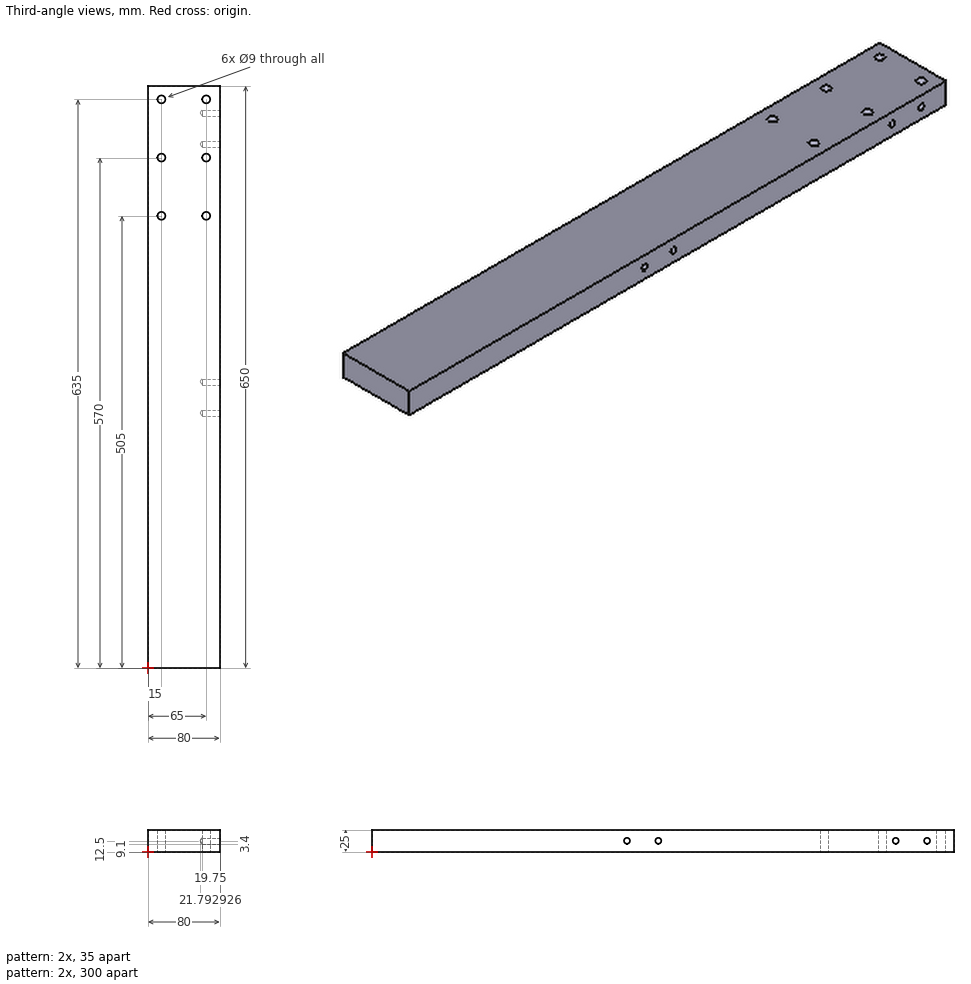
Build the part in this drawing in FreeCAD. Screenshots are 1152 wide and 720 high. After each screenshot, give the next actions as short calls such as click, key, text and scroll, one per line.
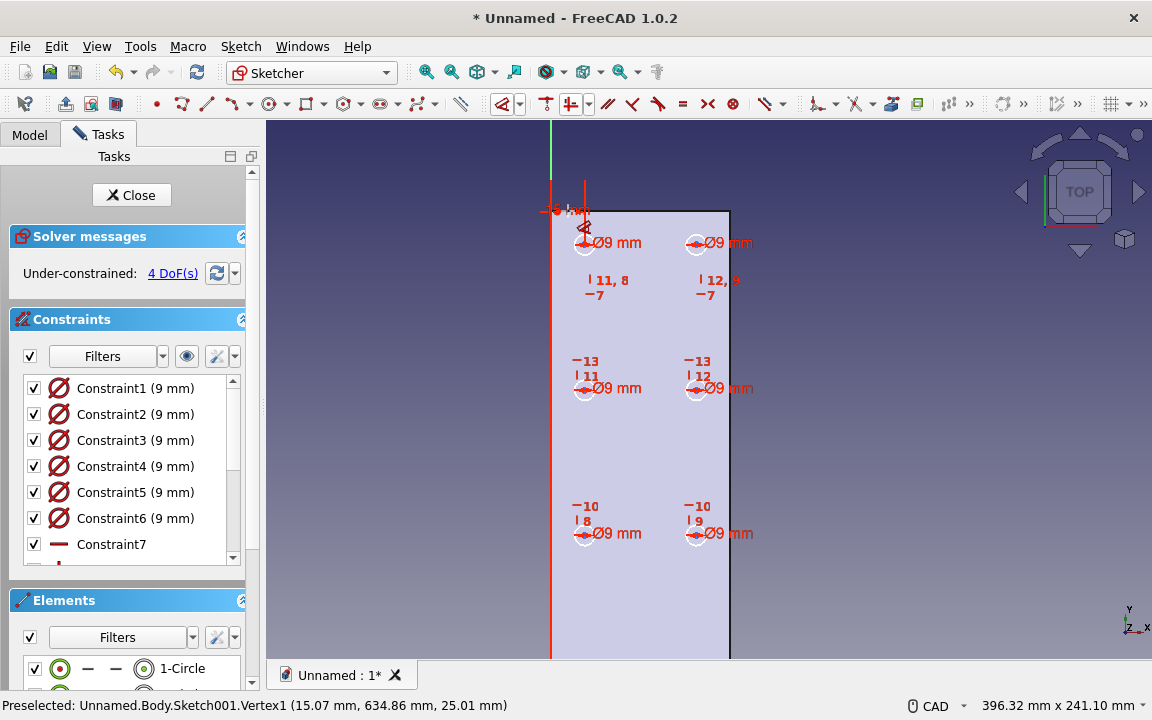
click(696, 245)
click(657, 211)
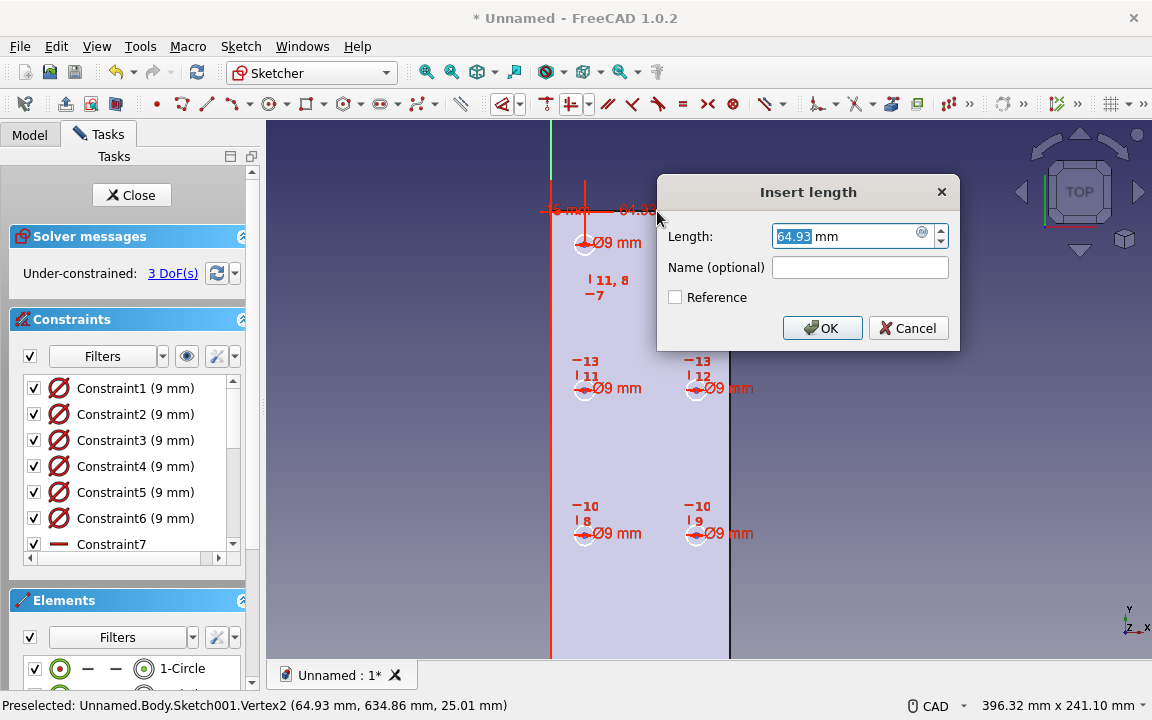
text(65)
key(Return)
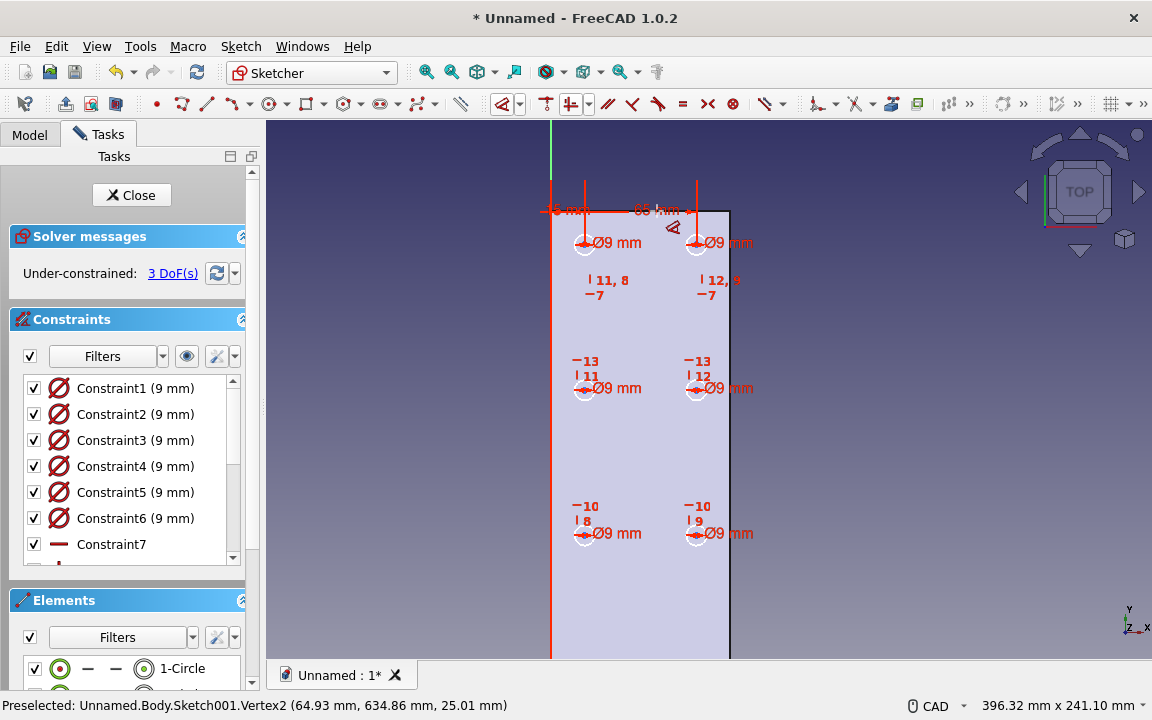
click(585, 245)
click(517, 438)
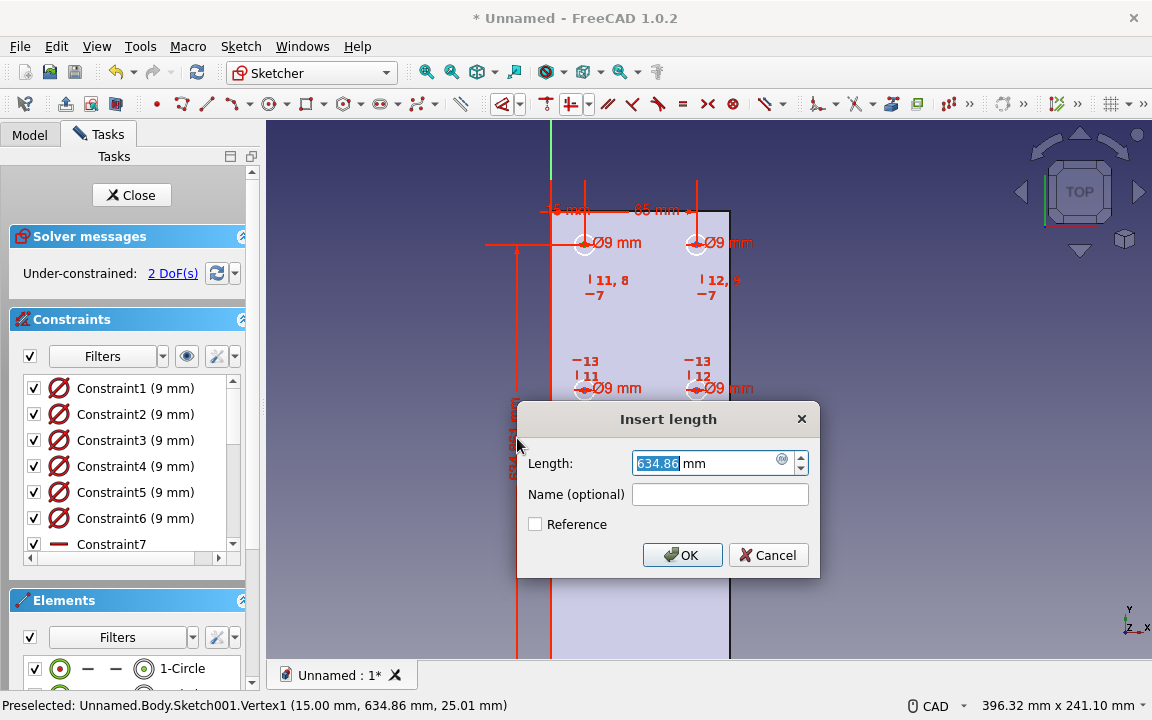
text(635)
key(Return)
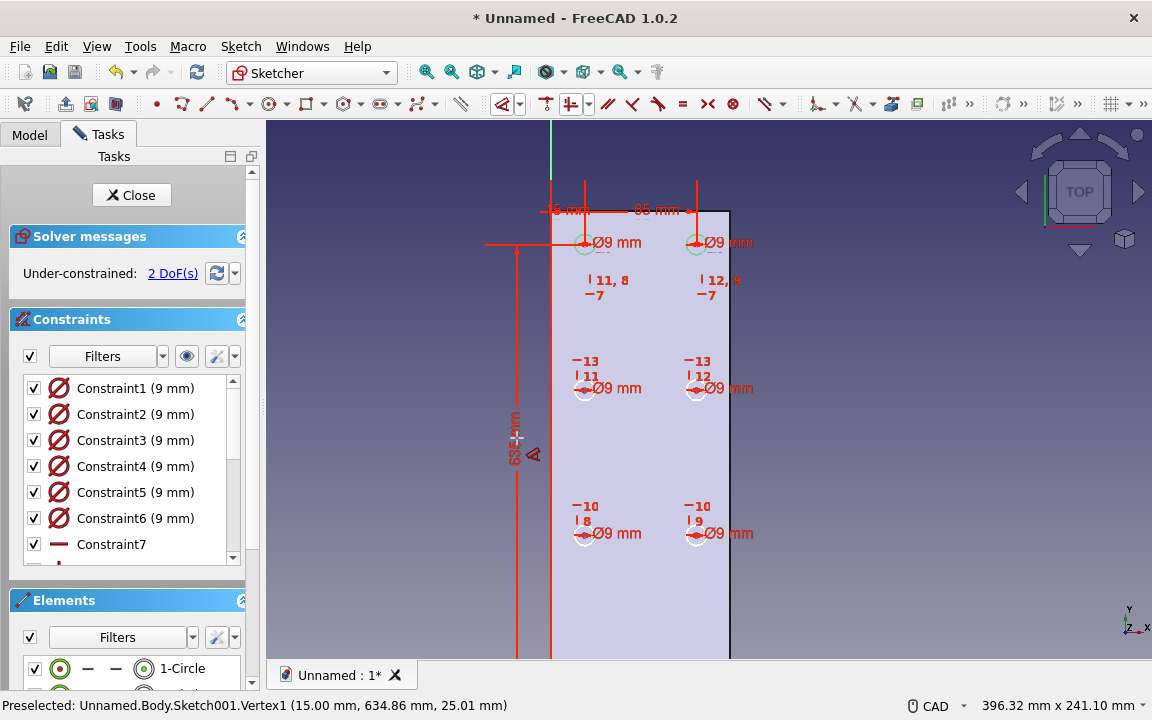
click(585, 535)
click(517, 583)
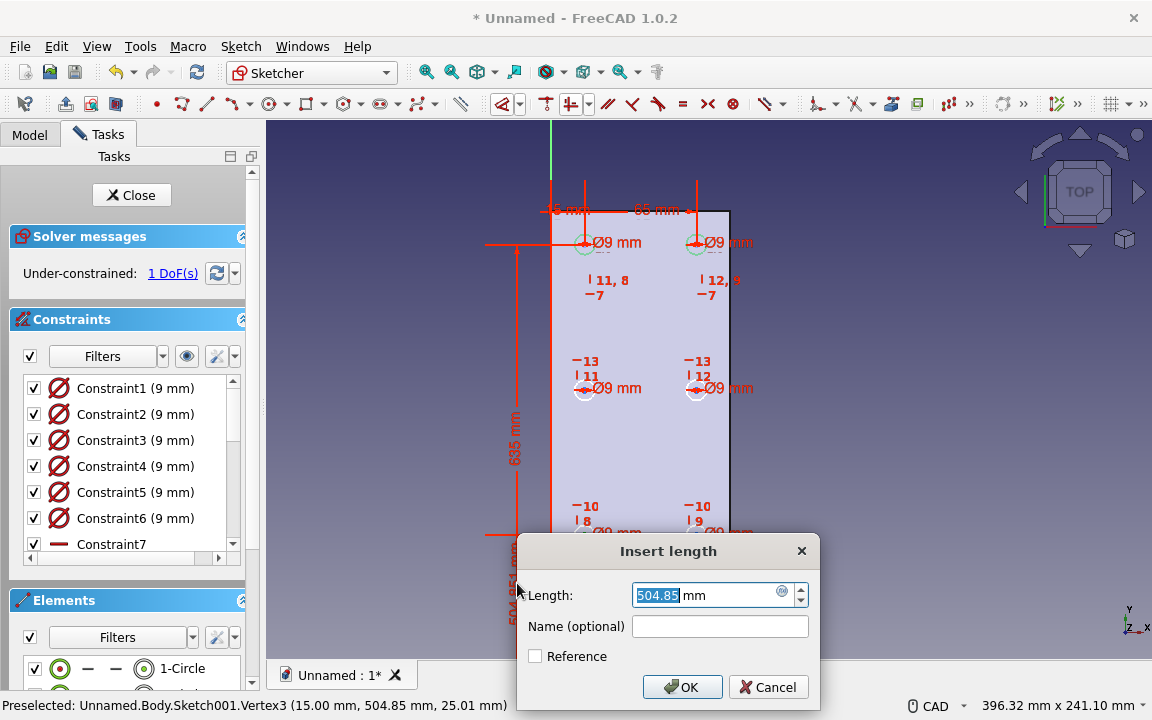
text(505)
key(Return)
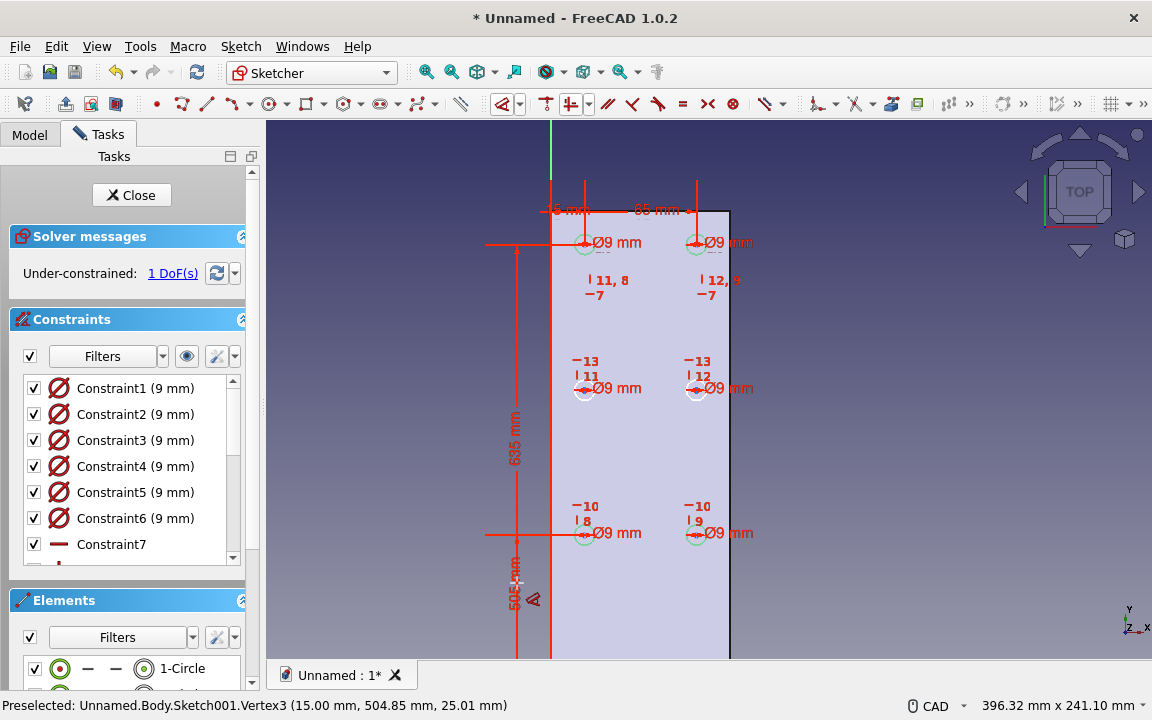
click(585, 390)
click(517, 511)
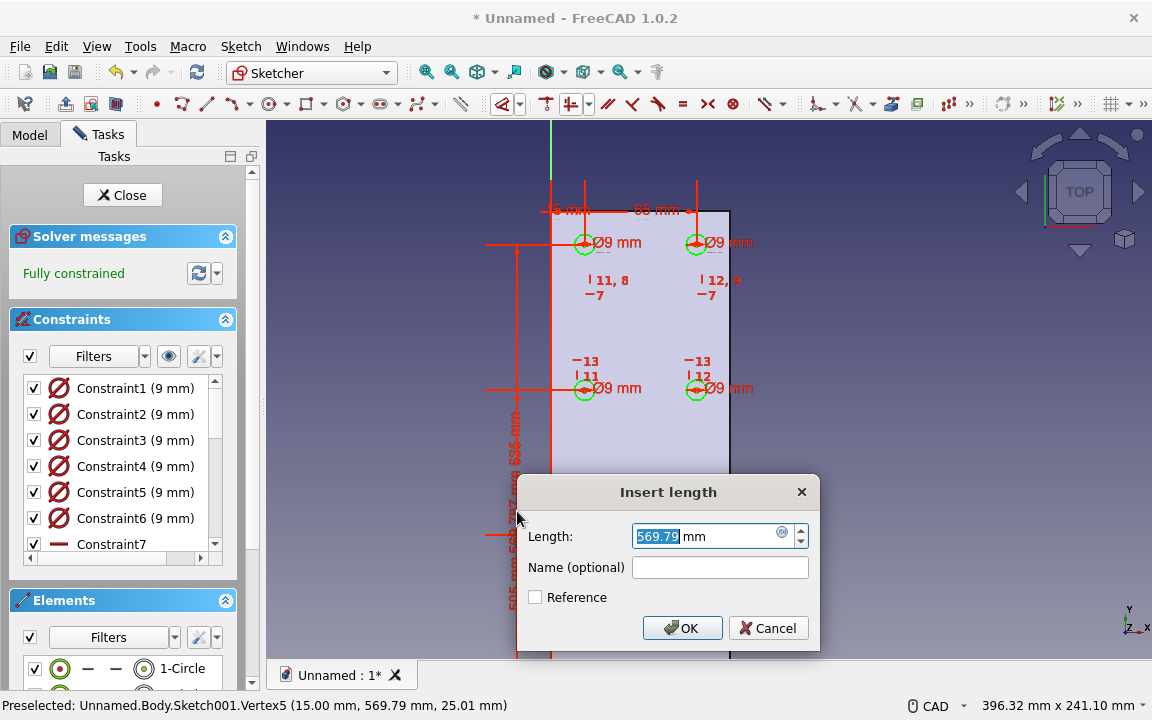
text(570)
key(Return)
key(Escape)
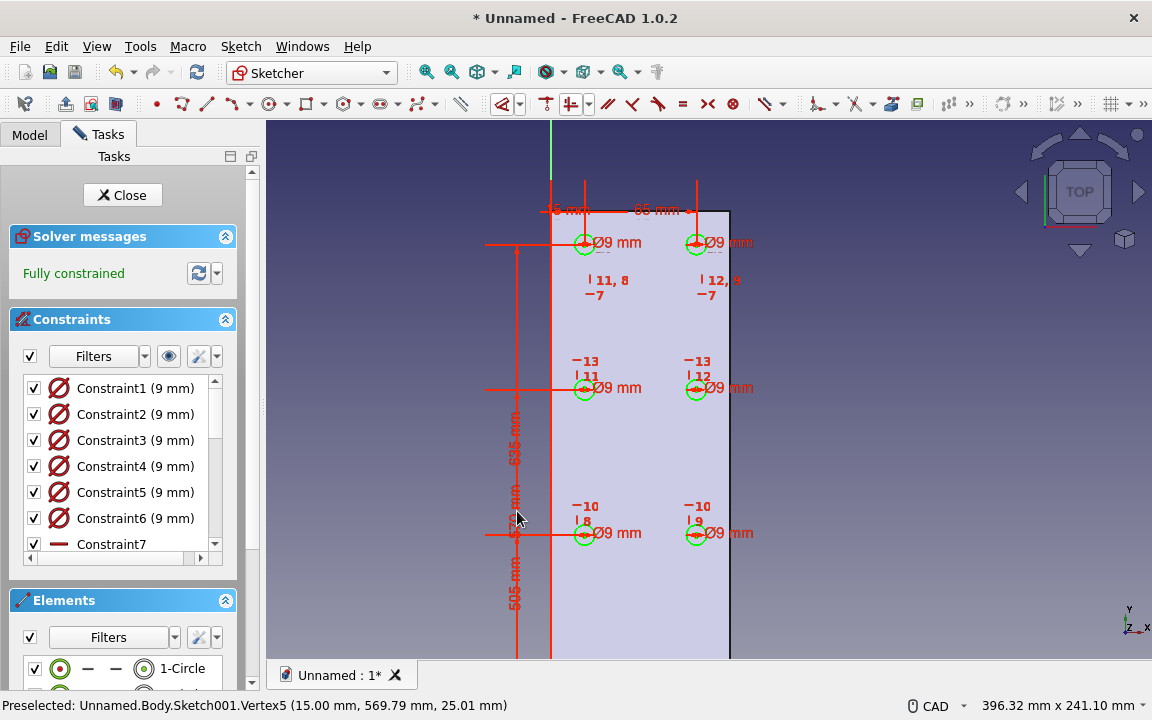
click(123, 195)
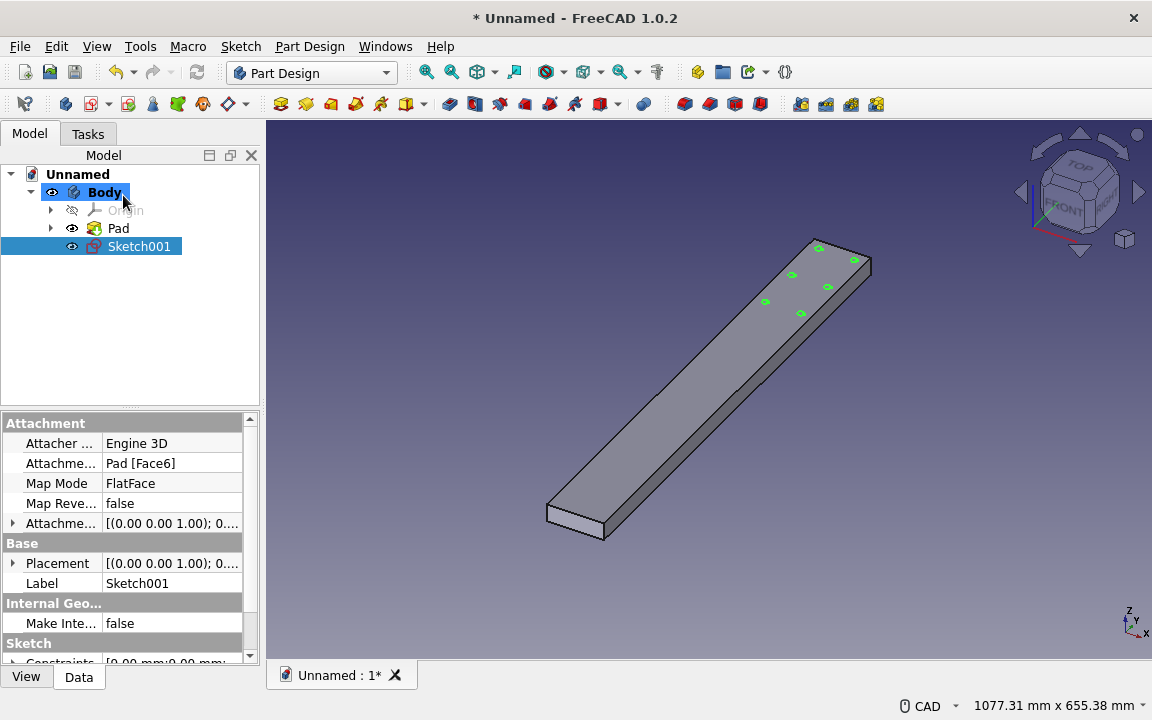
click(475, 104)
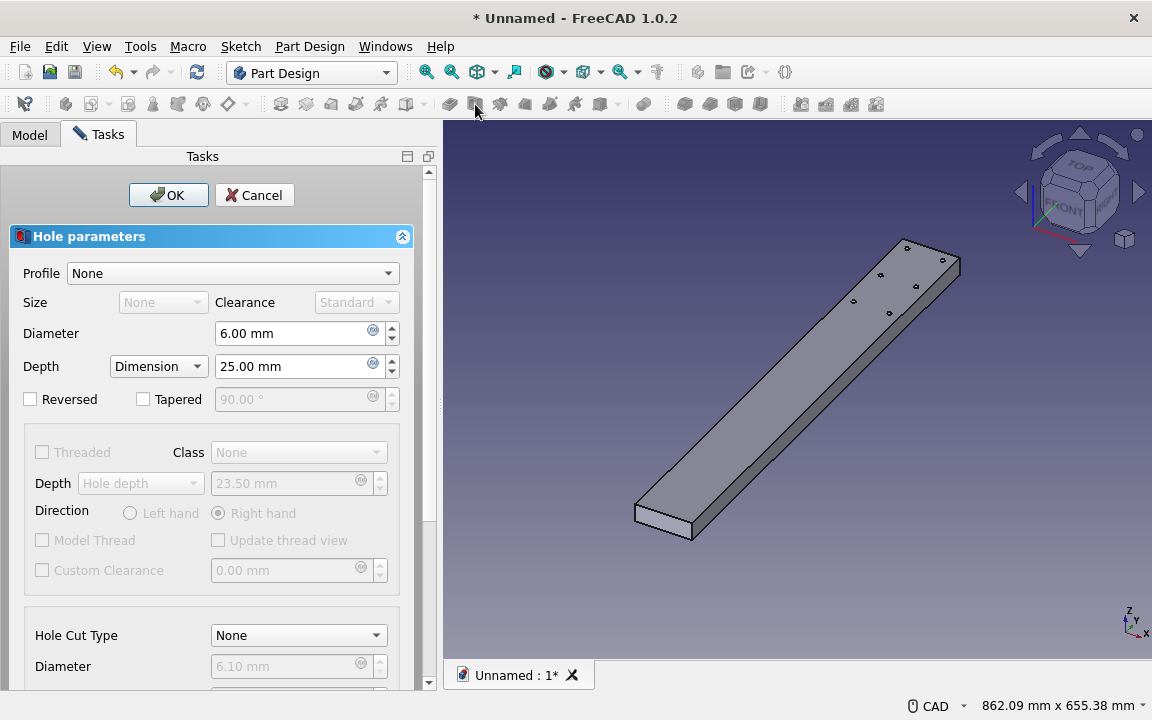
triple_click(300, 334)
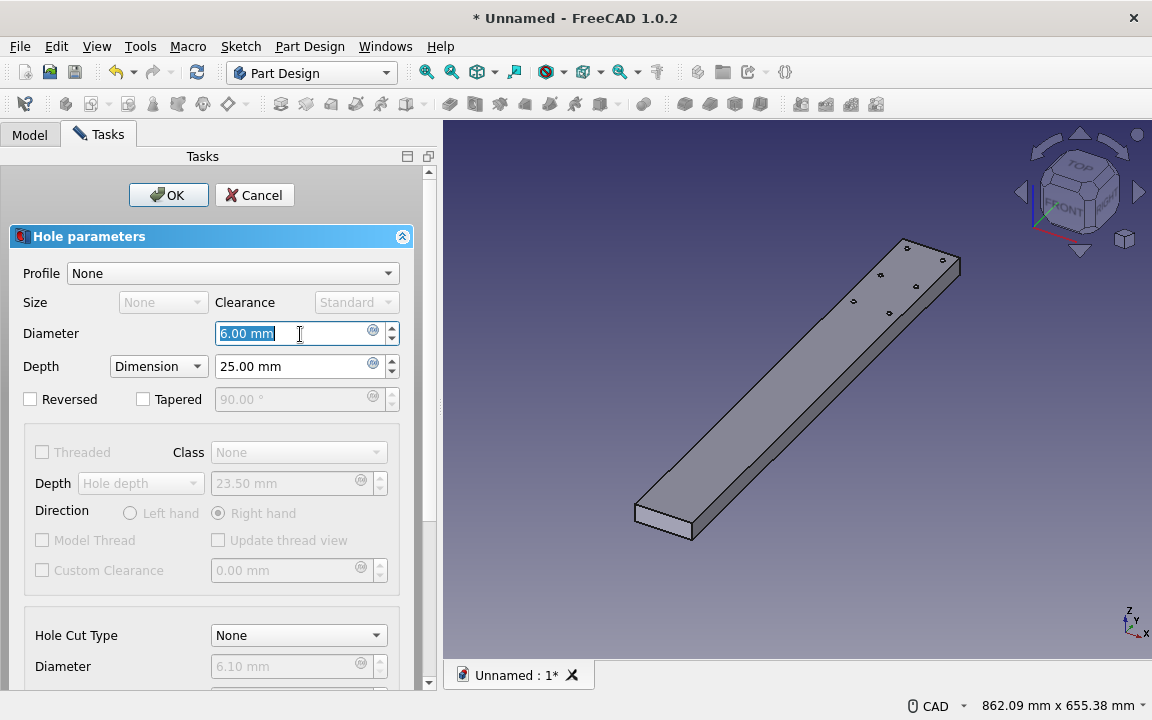
text(9)
key(Tab)